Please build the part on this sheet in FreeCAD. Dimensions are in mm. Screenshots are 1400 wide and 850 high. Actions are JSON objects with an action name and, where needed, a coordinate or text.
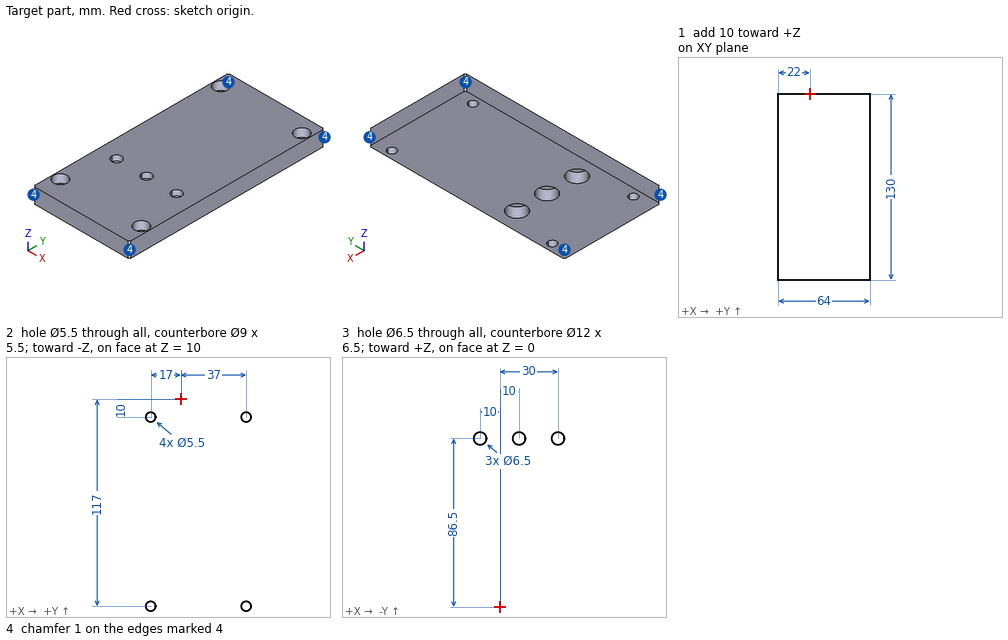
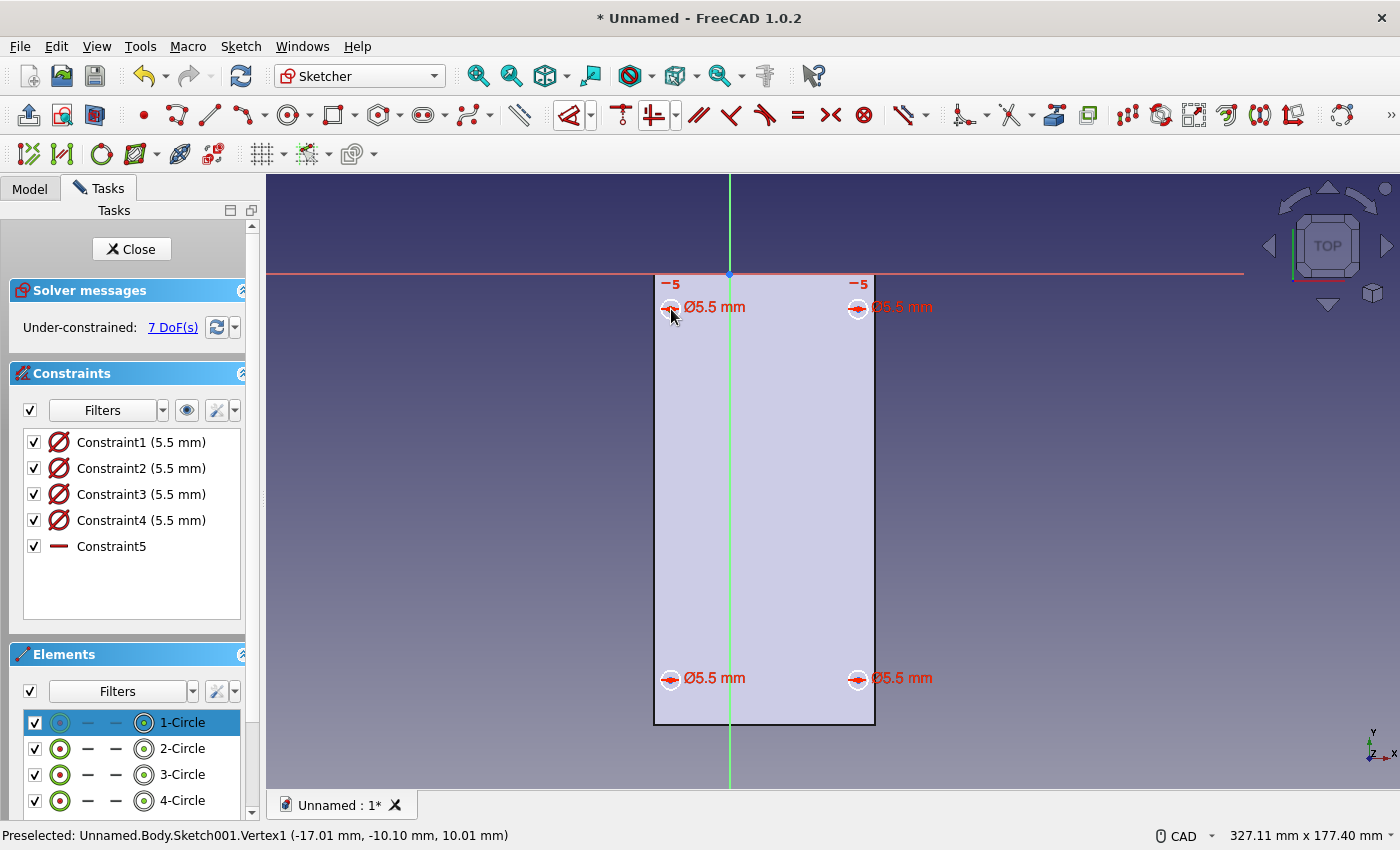
{"action": "left_click", "coordinate": [671, 680]}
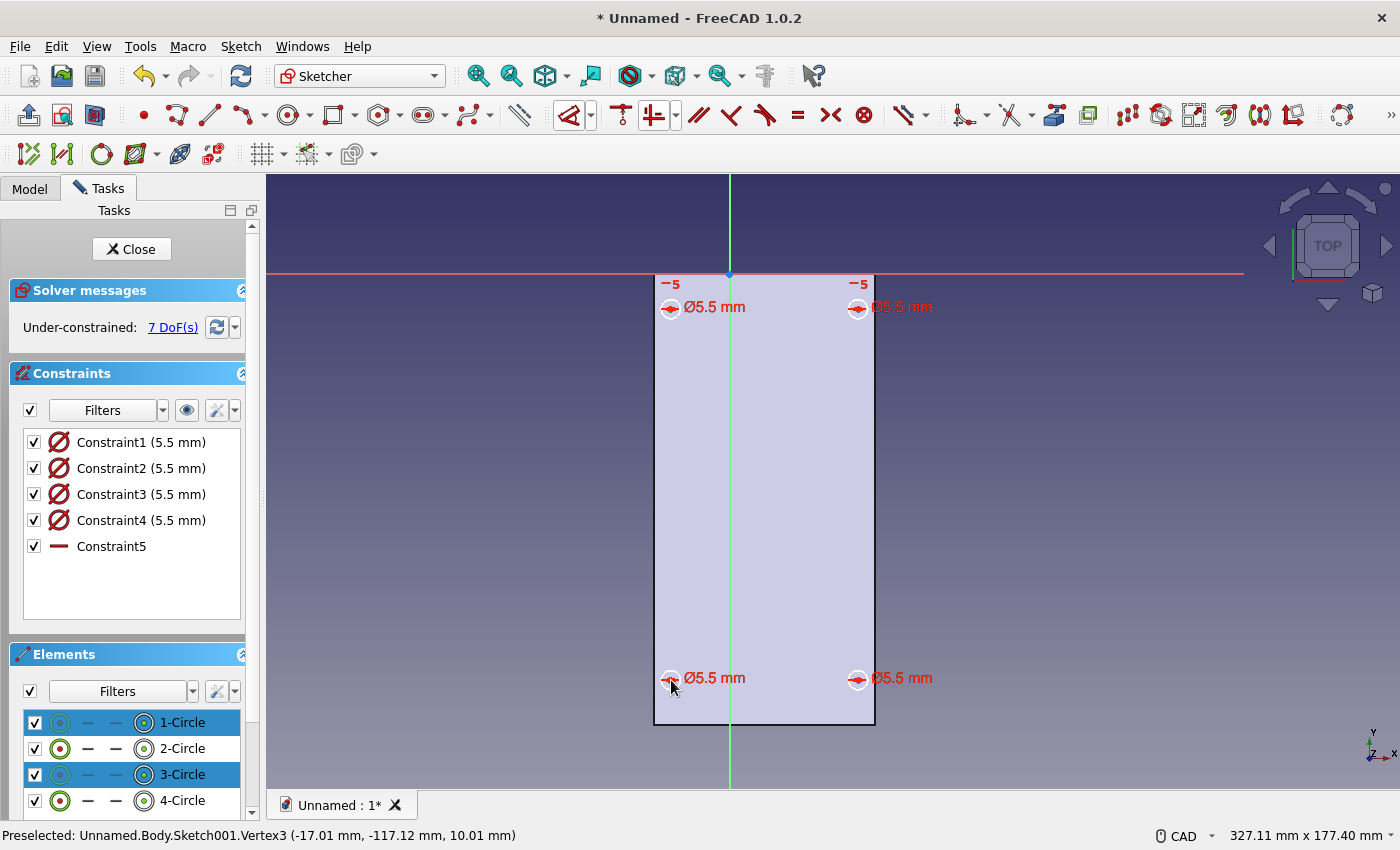
{"action": "key", "text": "v"}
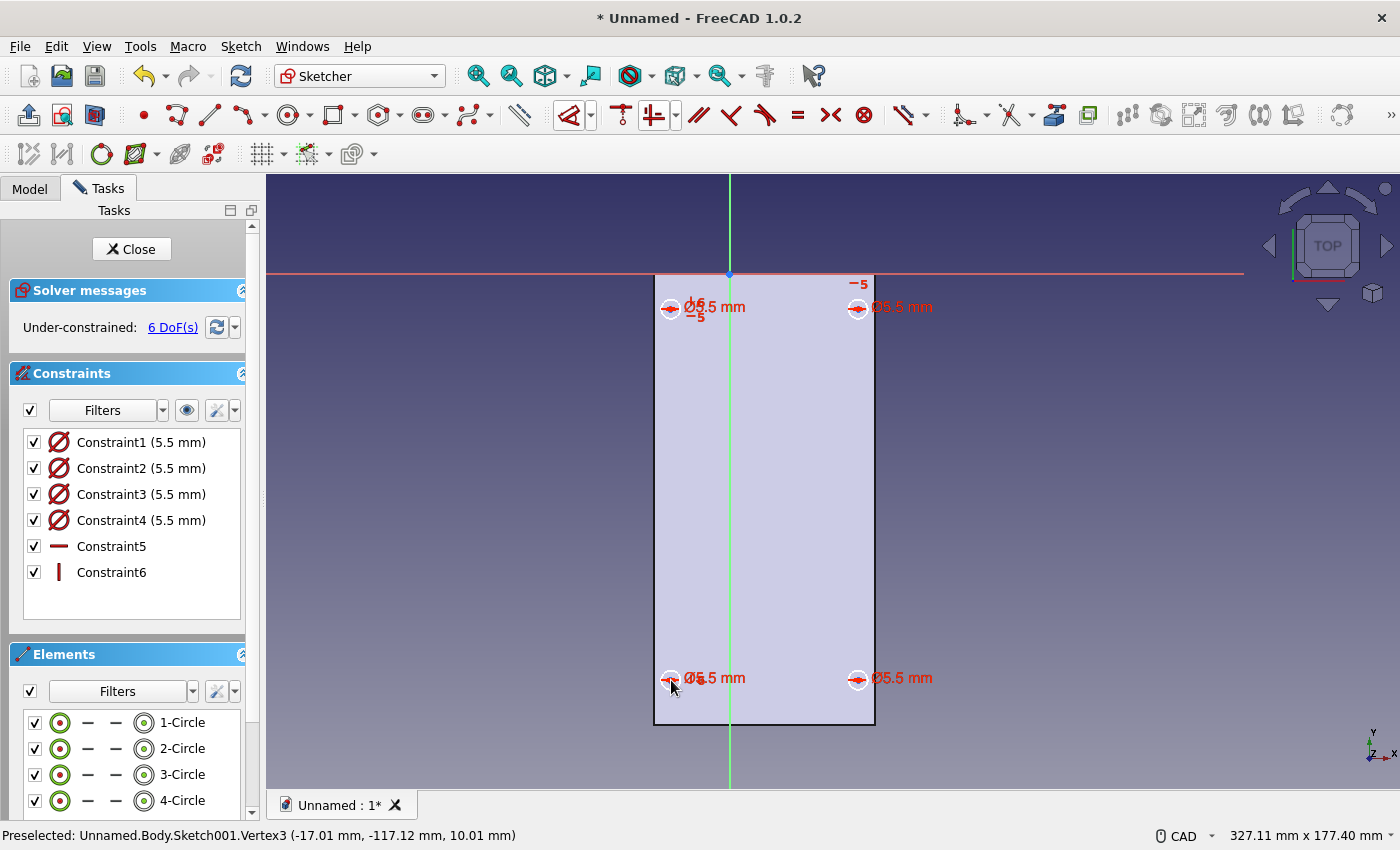
{"action": "left_click", "coordinate": [858, 309]}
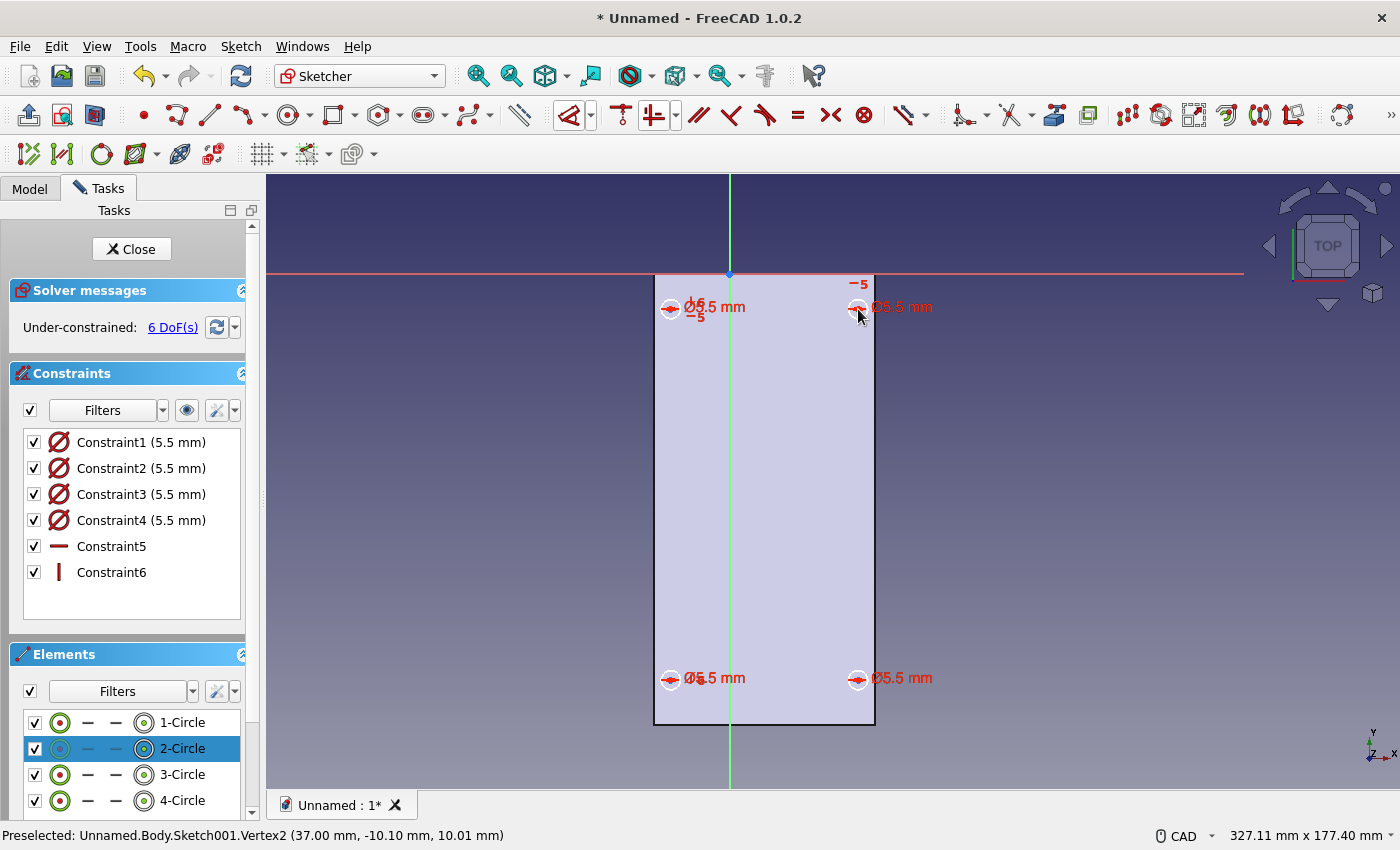
{"action": "left_click", "coordinate": [858, 680]}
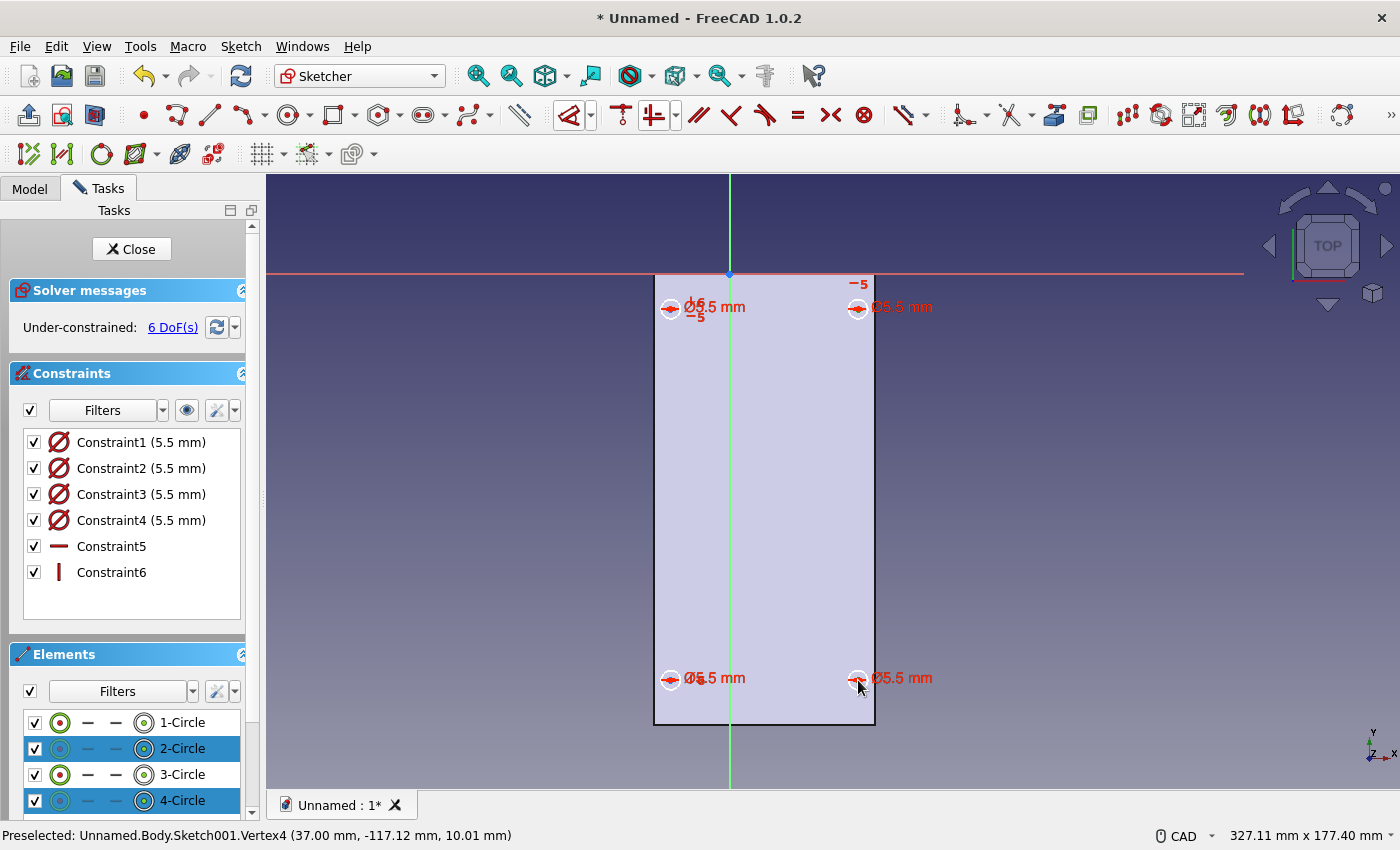
{"action": "left_click", "coordinate": [676, 116]}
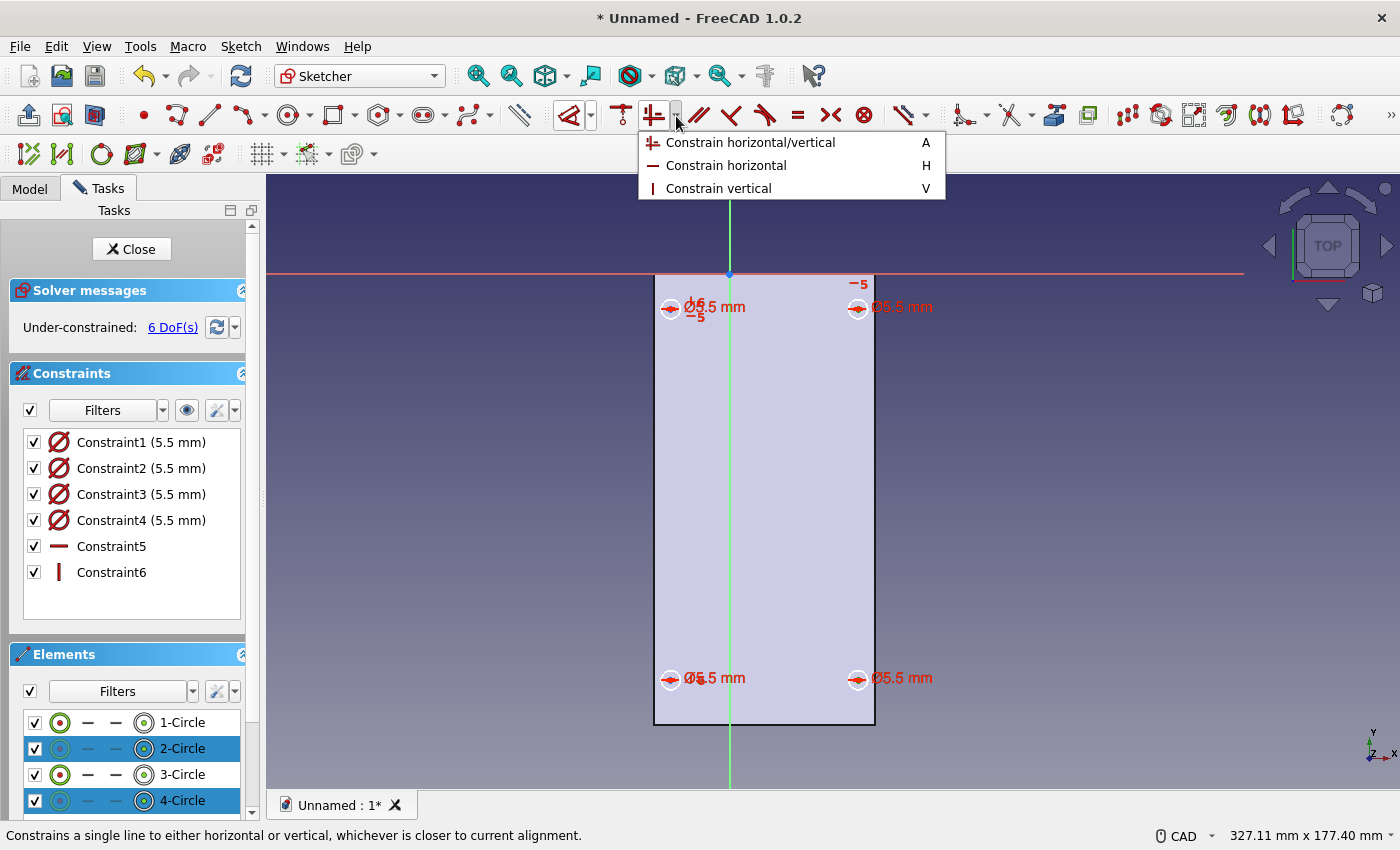
{"action": "left_click", "coordinate": [792, 188]}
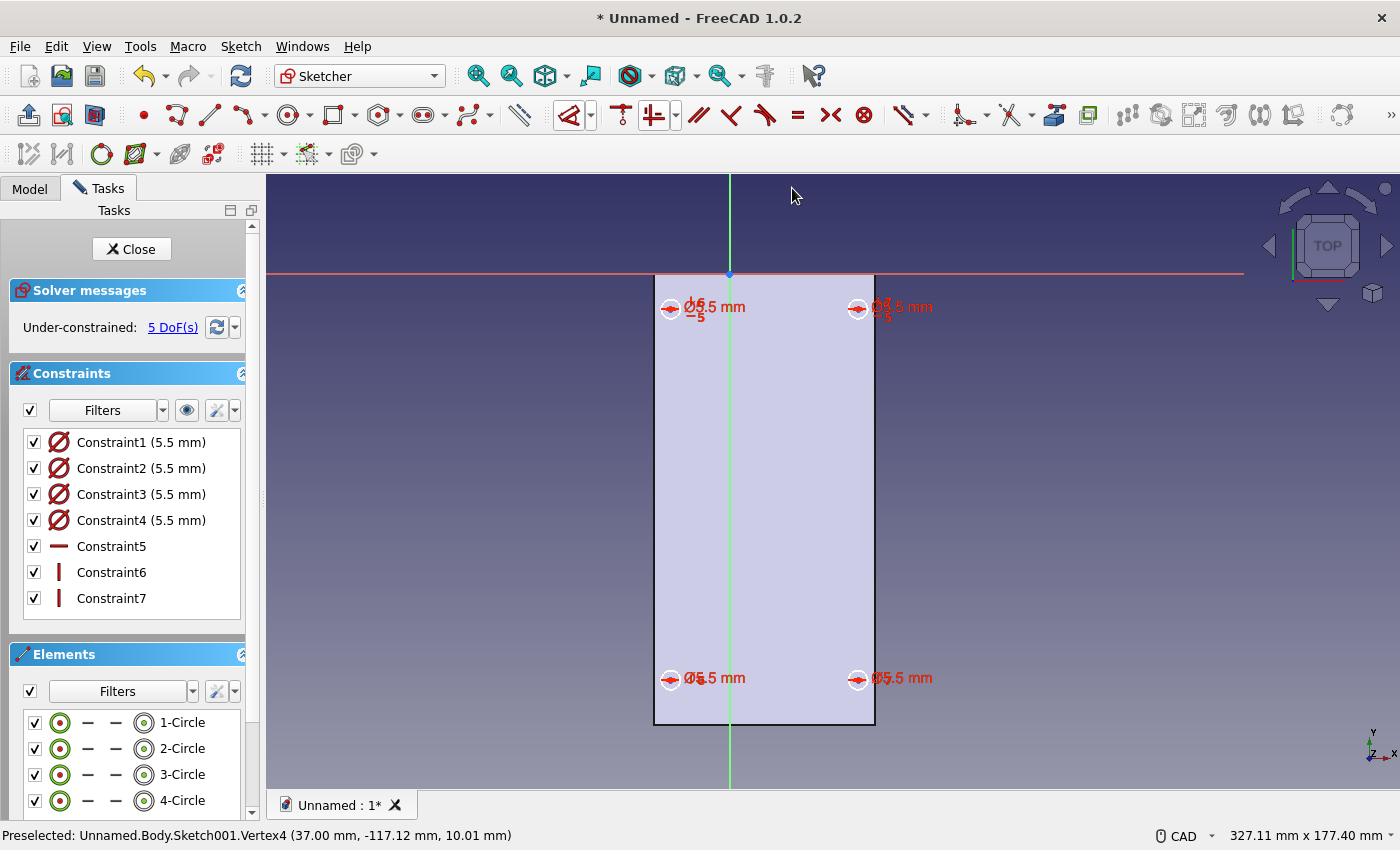
{"action": "left_click", "coordinate": [671, 680]}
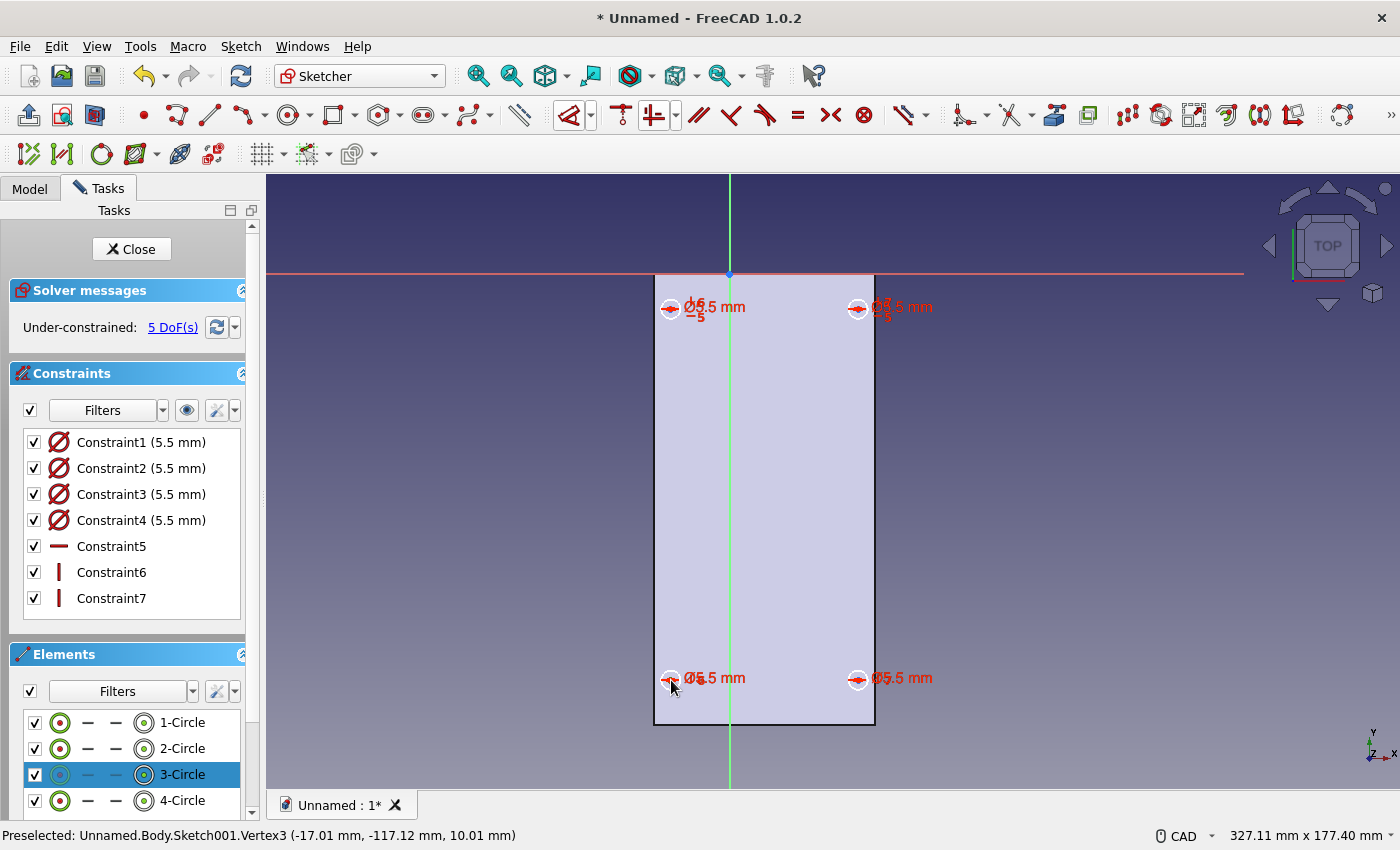
{"action": "left_click", "coordinate": [858, 680]}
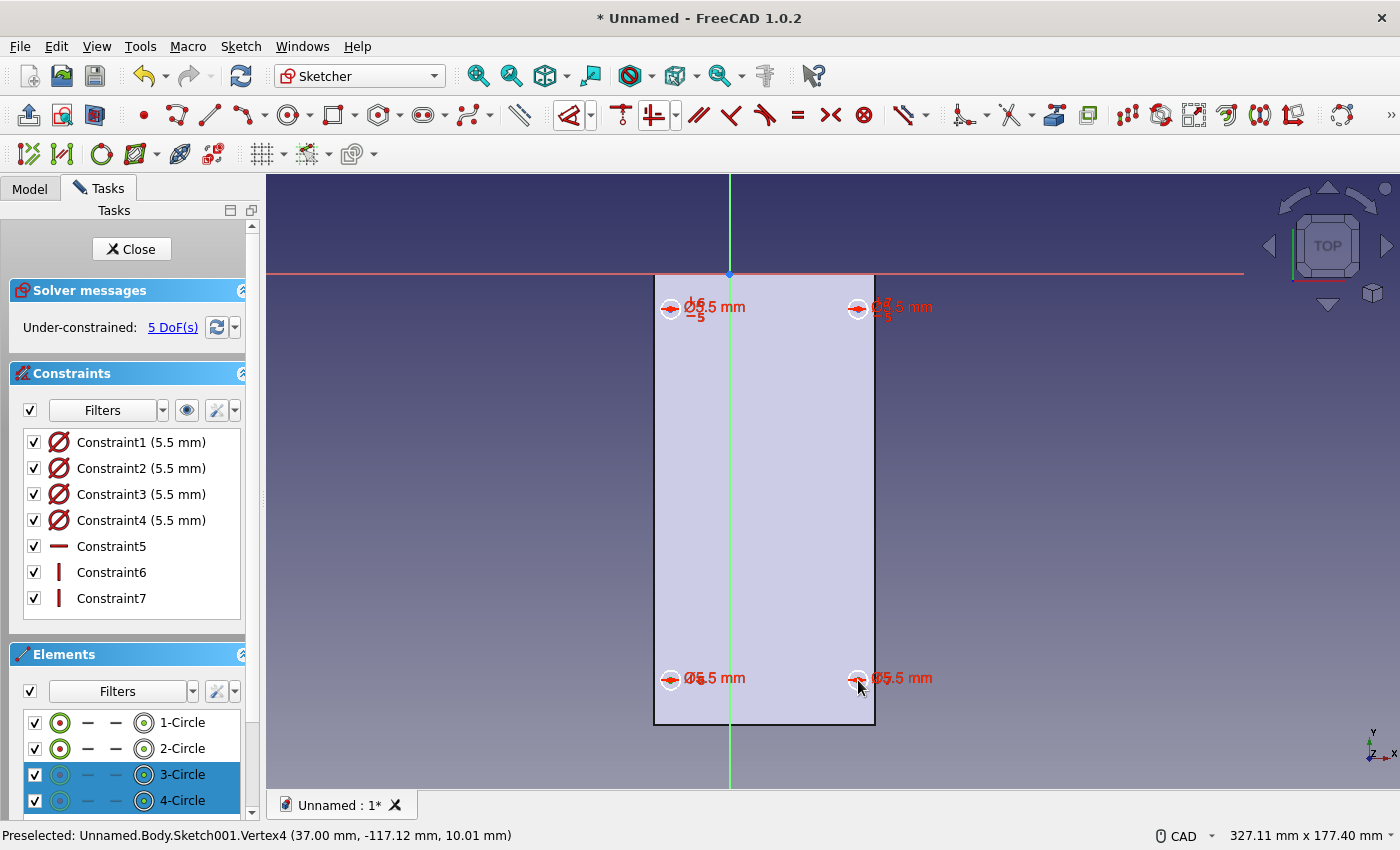
{"action": "key", "text": "h"}